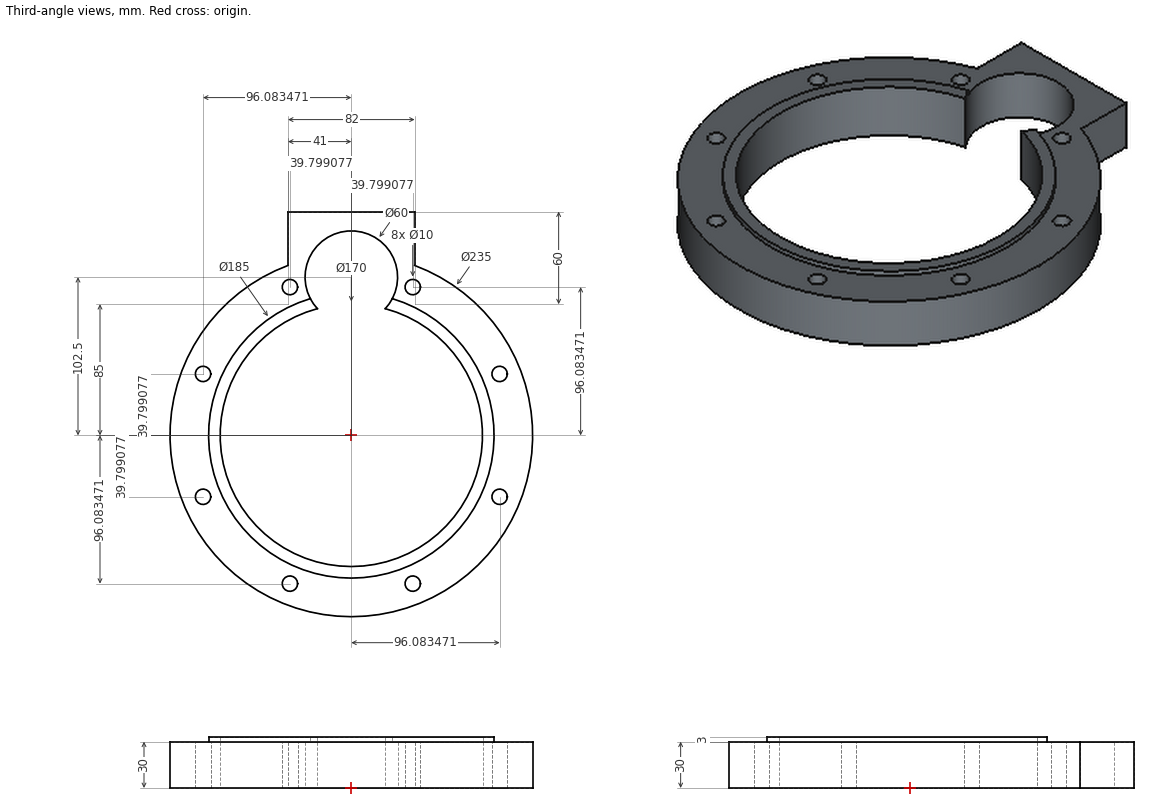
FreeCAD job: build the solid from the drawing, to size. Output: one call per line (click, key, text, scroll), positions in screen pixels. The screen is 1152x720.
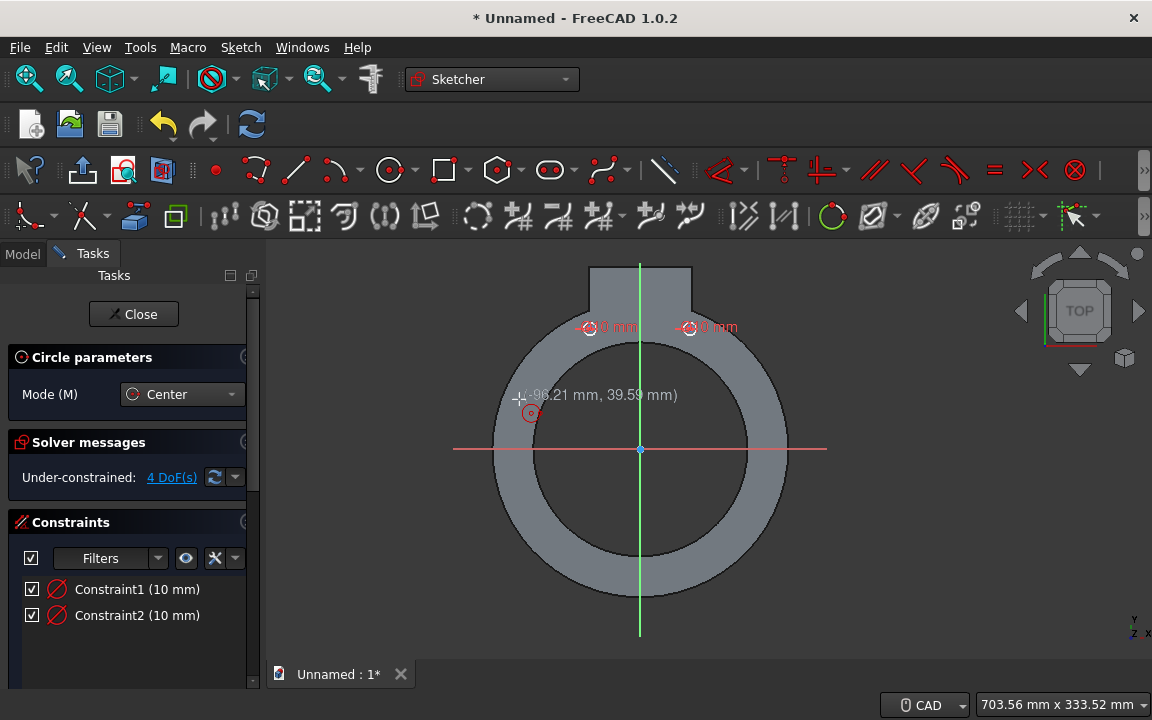
click(519, 399)
move(524, 395)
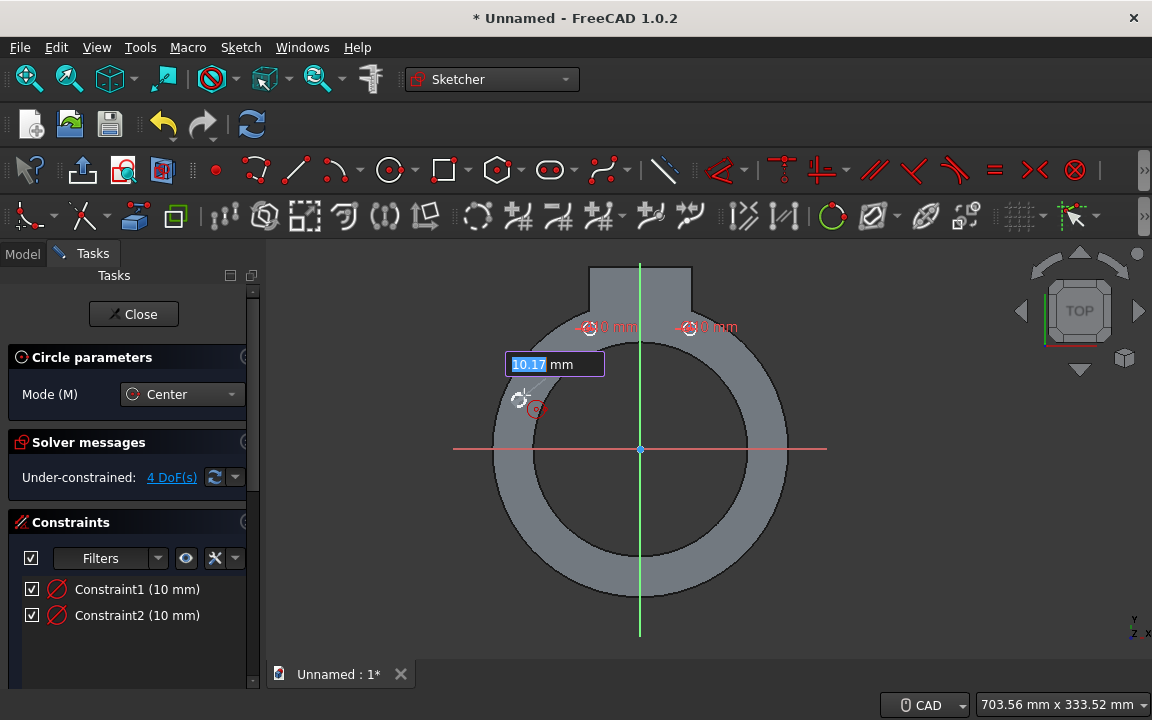
text(10)
key(Return)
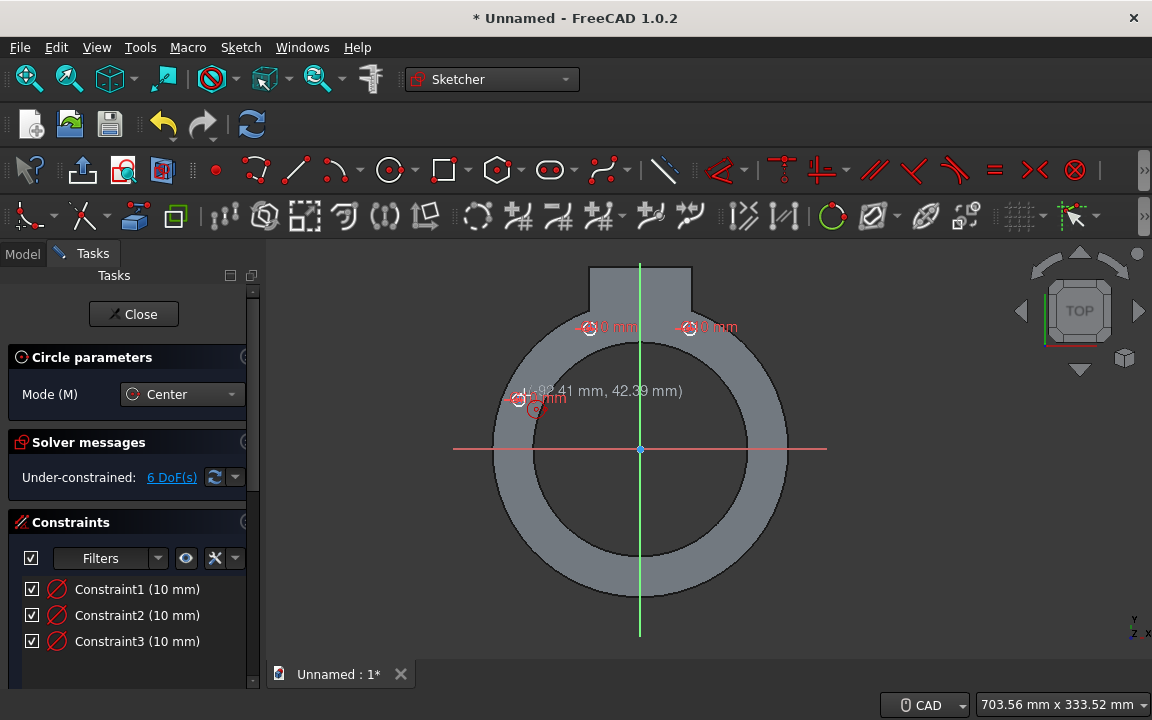
scroll(519, 500, up, 7)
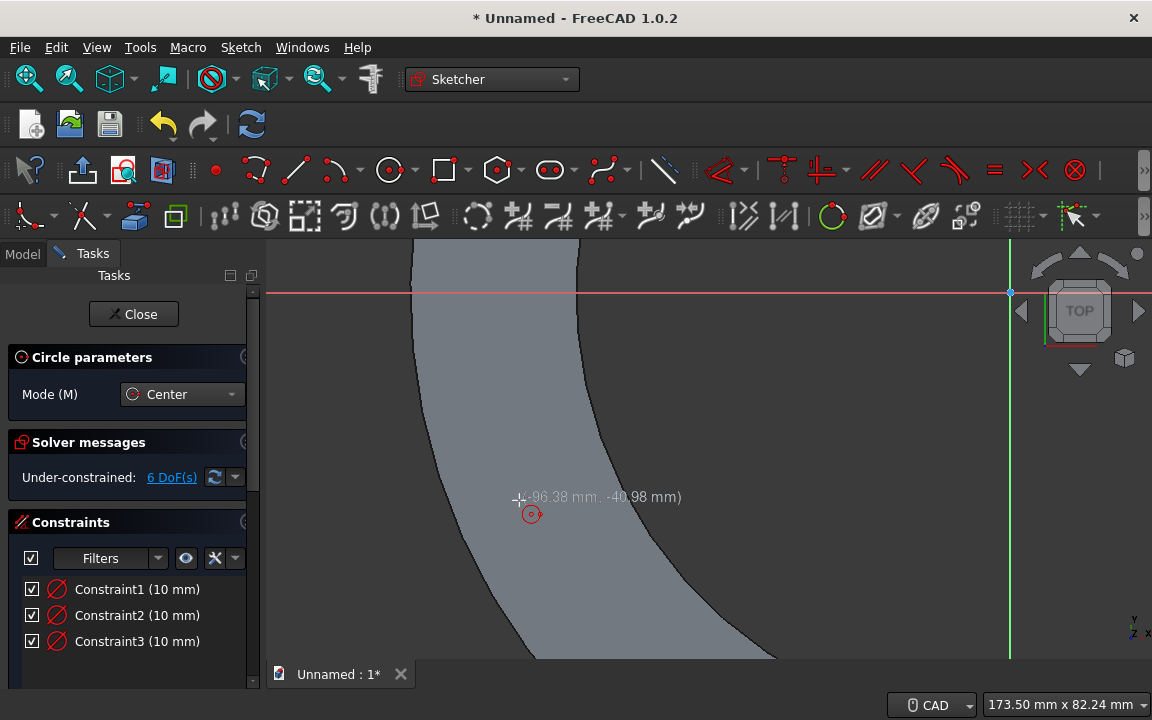
scroll(519, 500, down, 7)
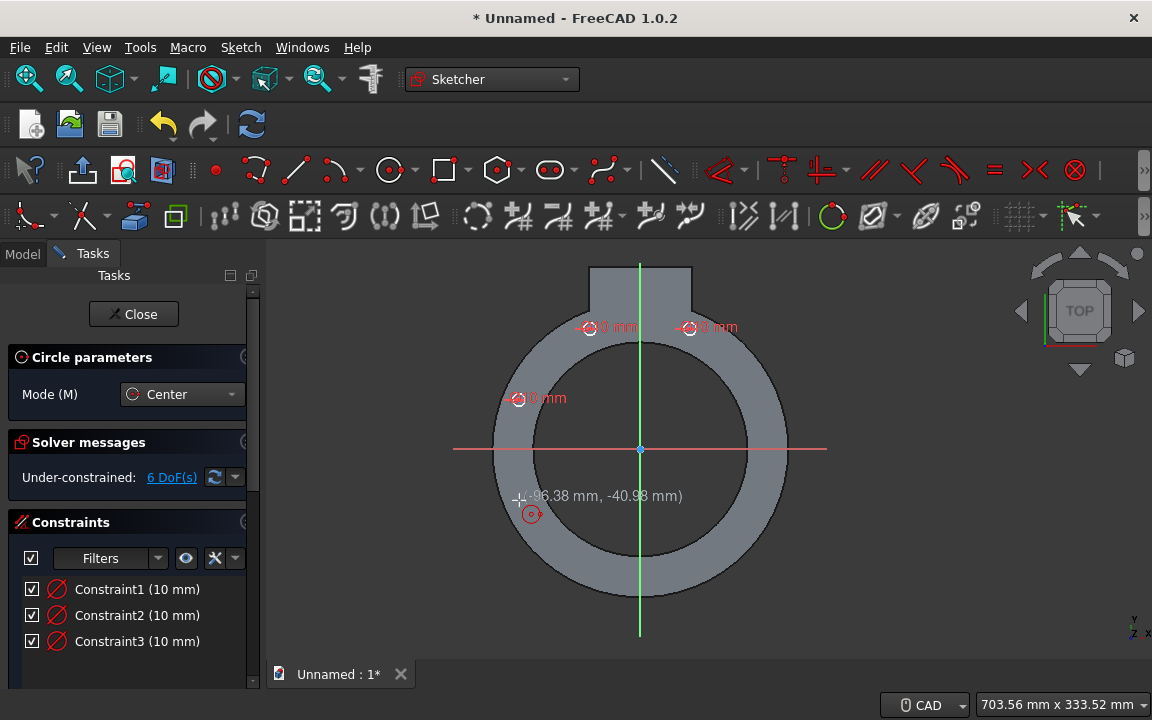
click(519, 500)
move(524, 495)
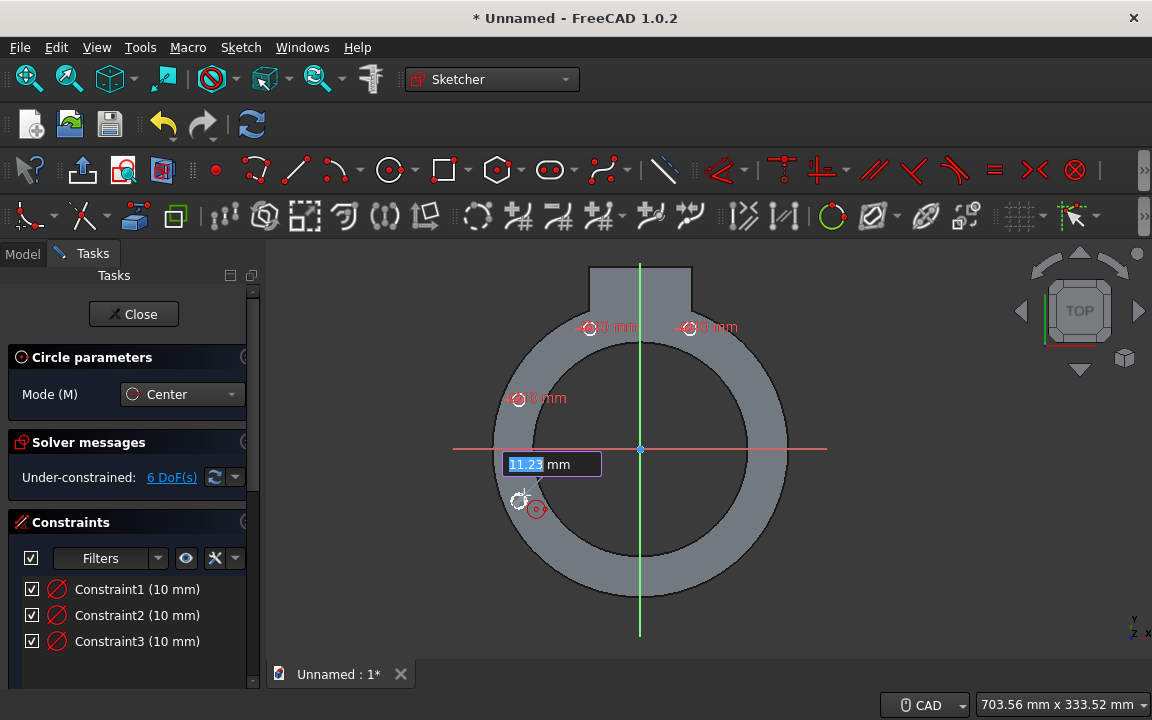
text(10)
key(Return)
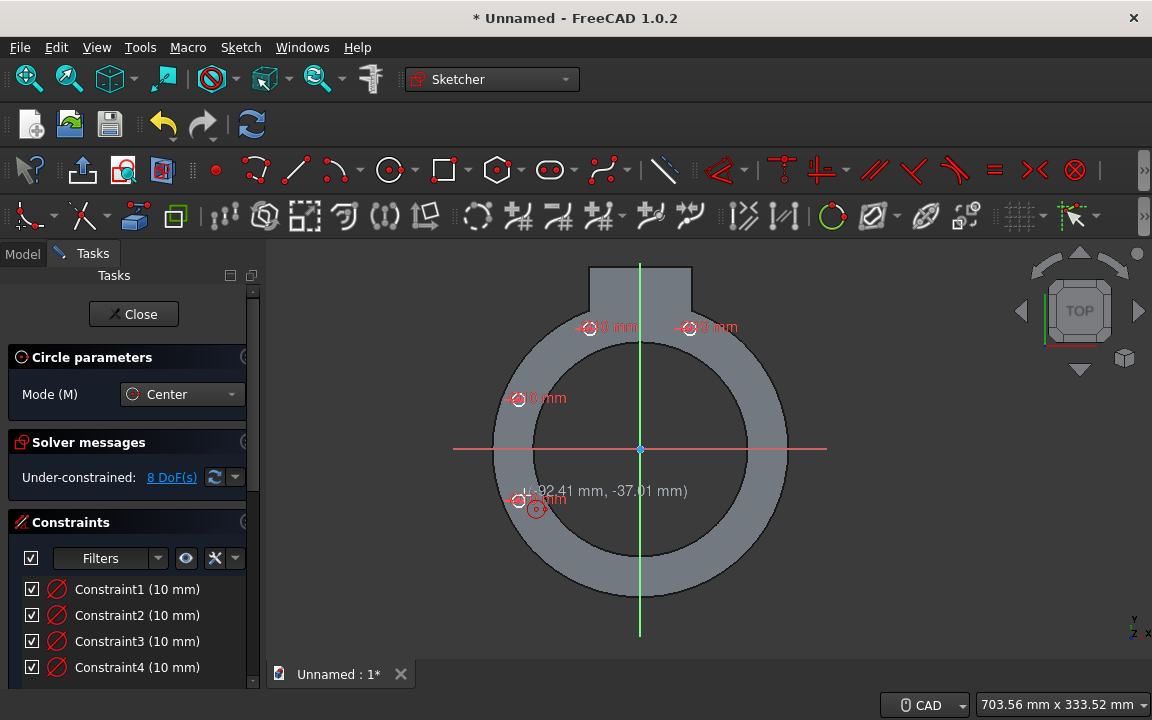
scroll(590, 570, up, 7)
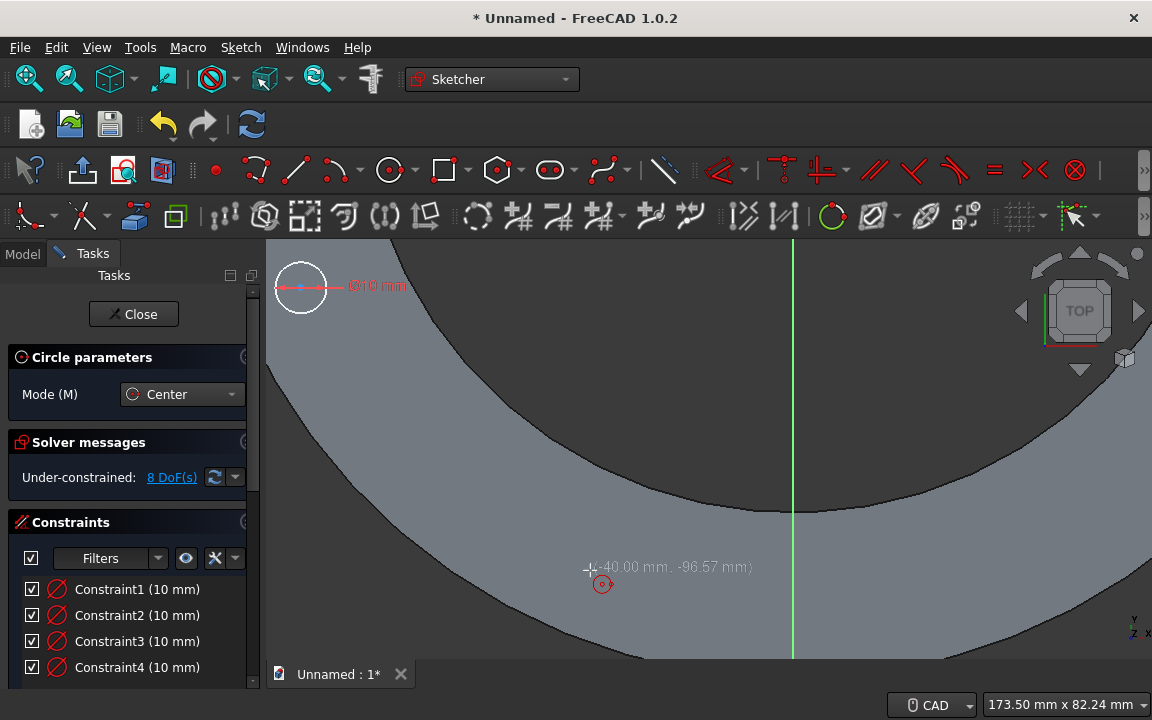
scroll(591, 570, down, 7)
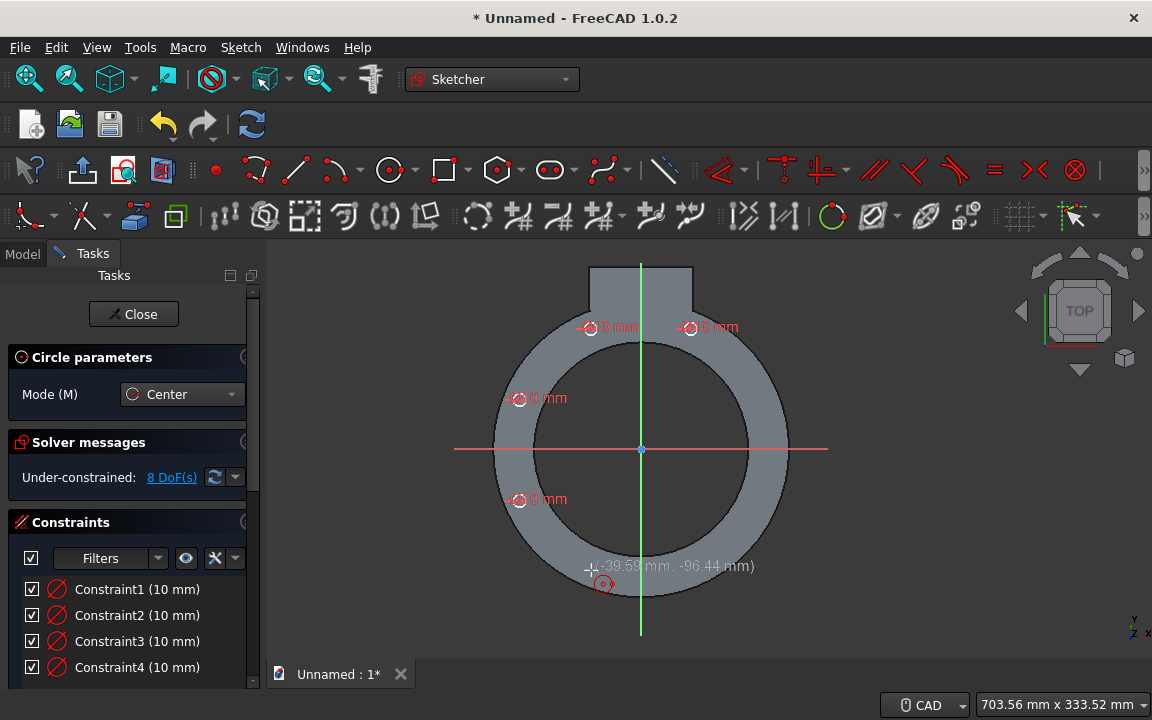
click(591, 570)
move(595, 566)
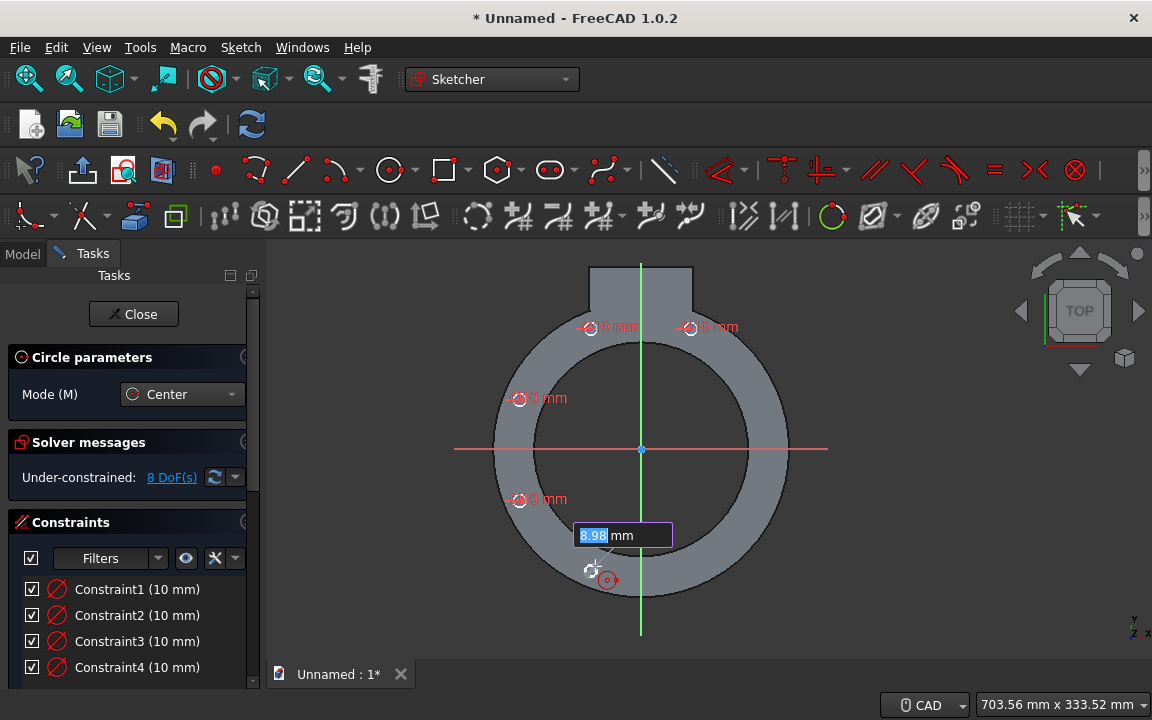
text(10)
key(Return)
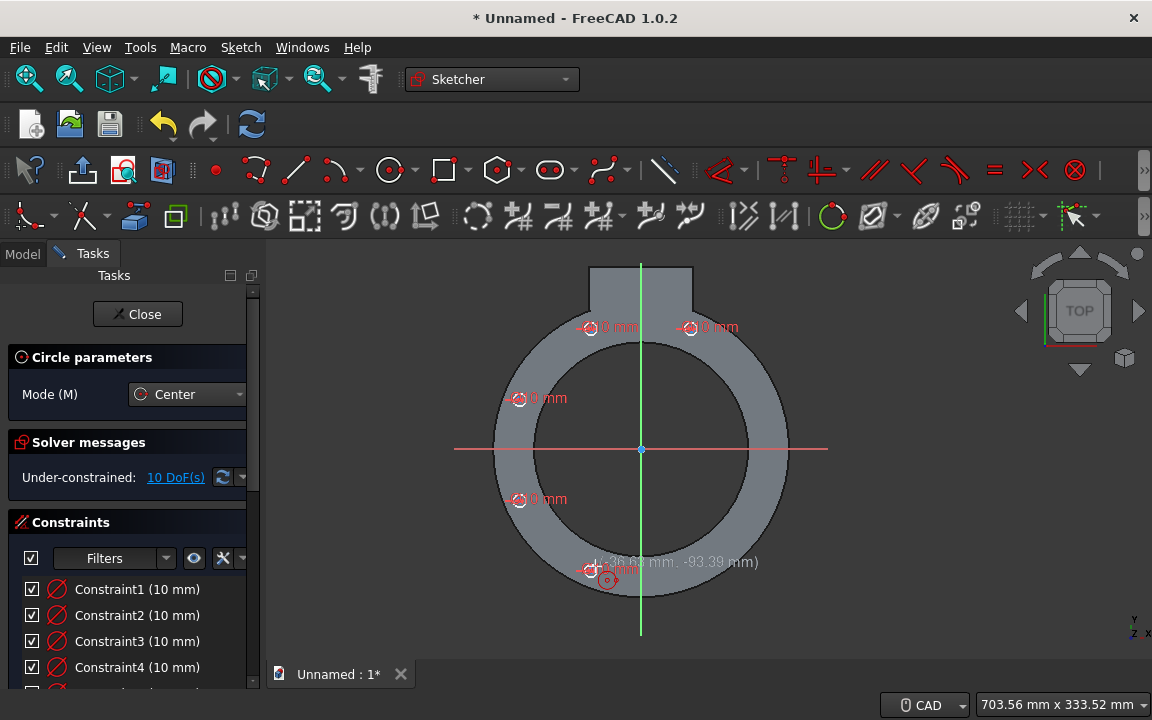
scroll(691, 570, up, 7)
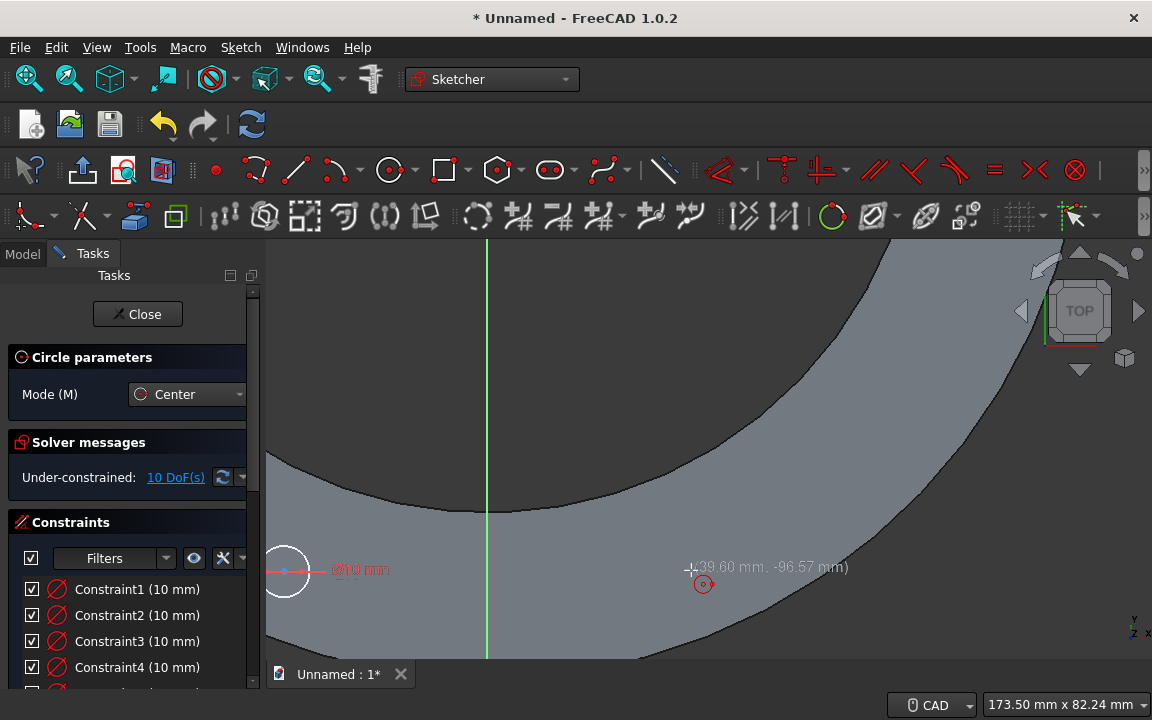
scroll(691, 570, down, 7)